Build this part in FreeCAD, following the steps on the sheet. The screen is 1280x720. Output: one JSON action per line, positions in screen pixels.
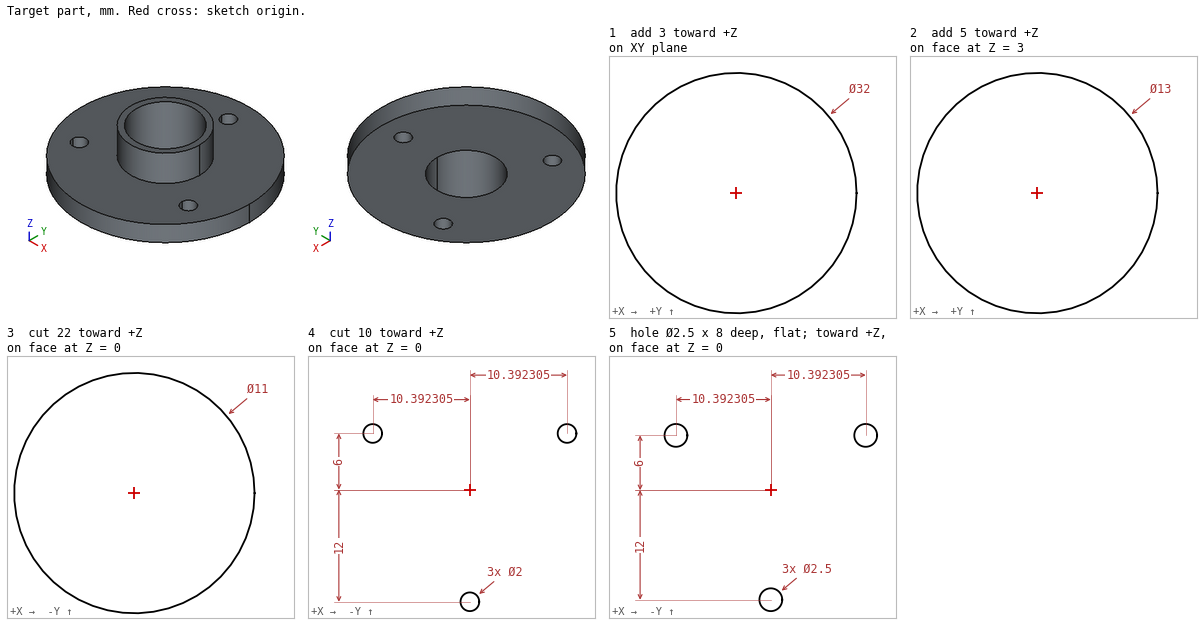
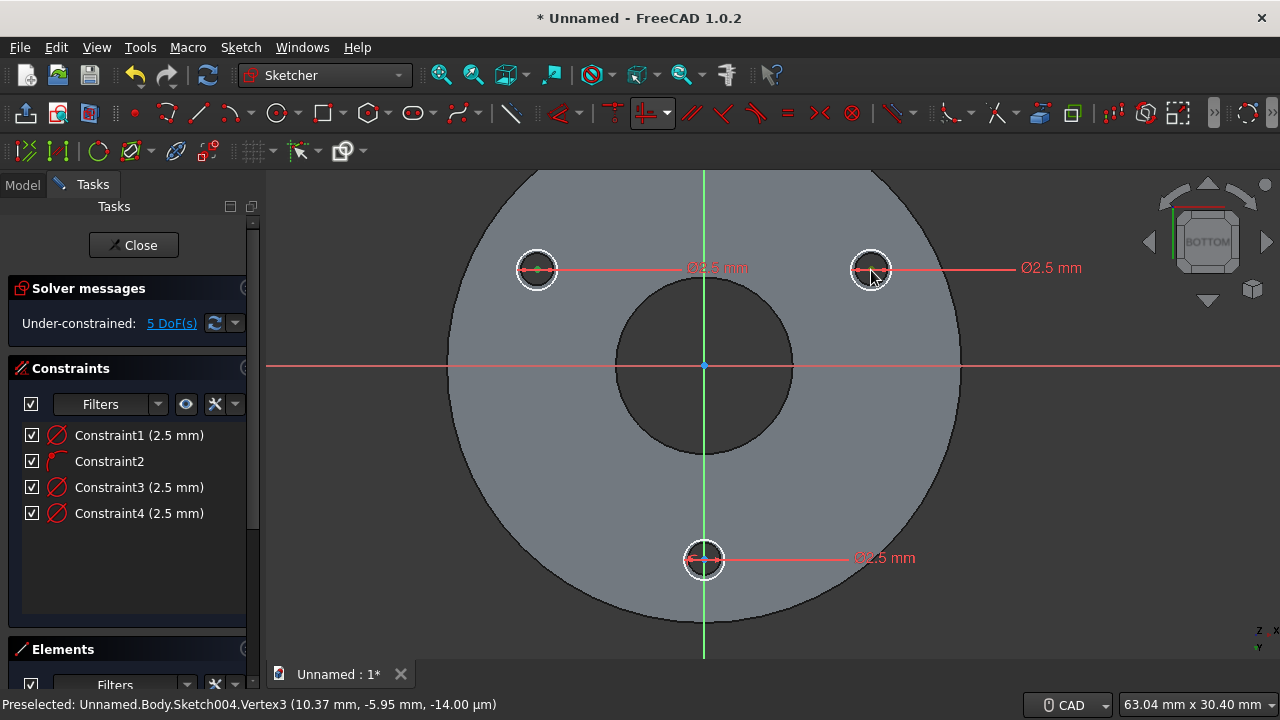
{"action": "key", "text": "h"}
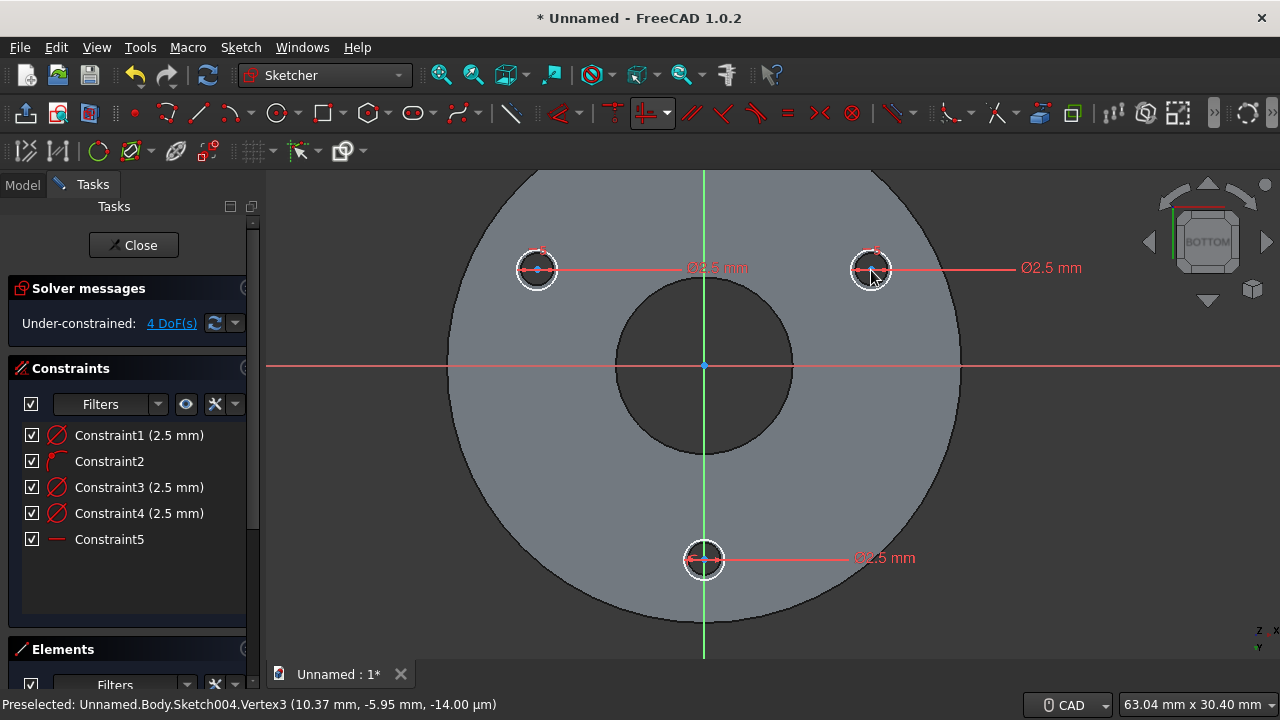
{"action": "left_click", "coordinate": [558, 114]}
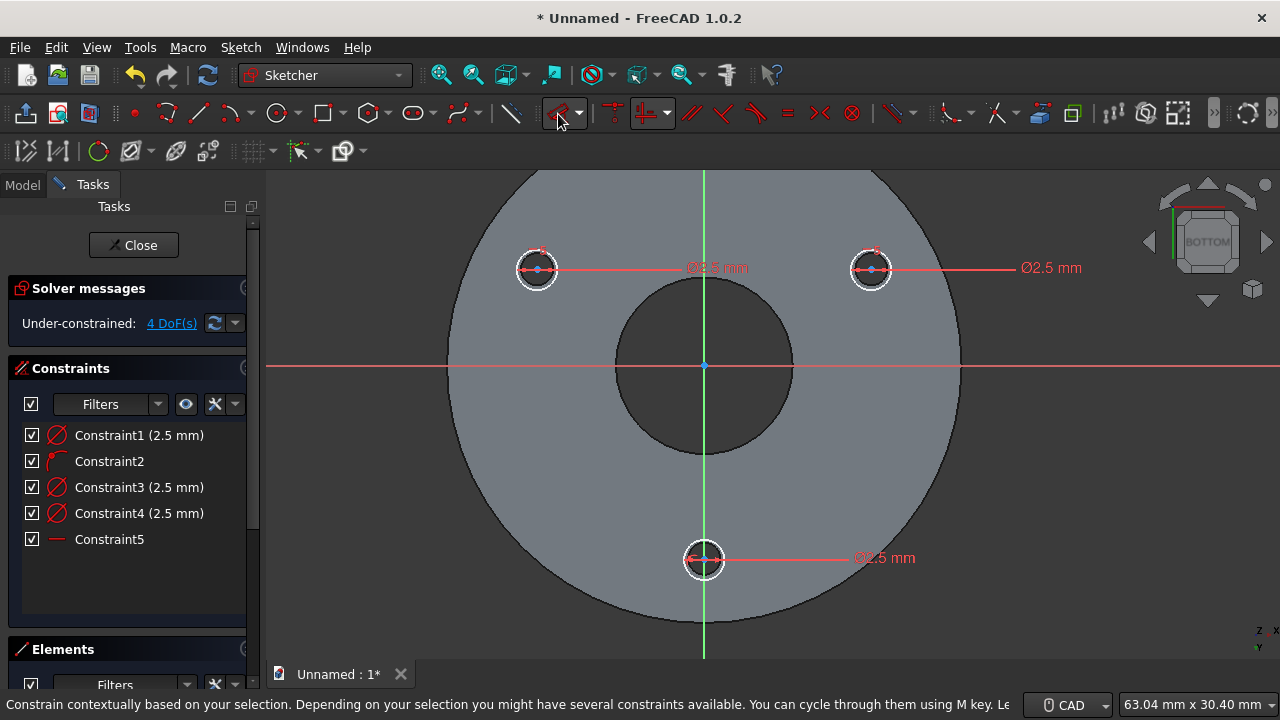
{"action": "left_click", "coordinate": [537, 270]}
{"action": "left_click", "coordinate": [503, 318]}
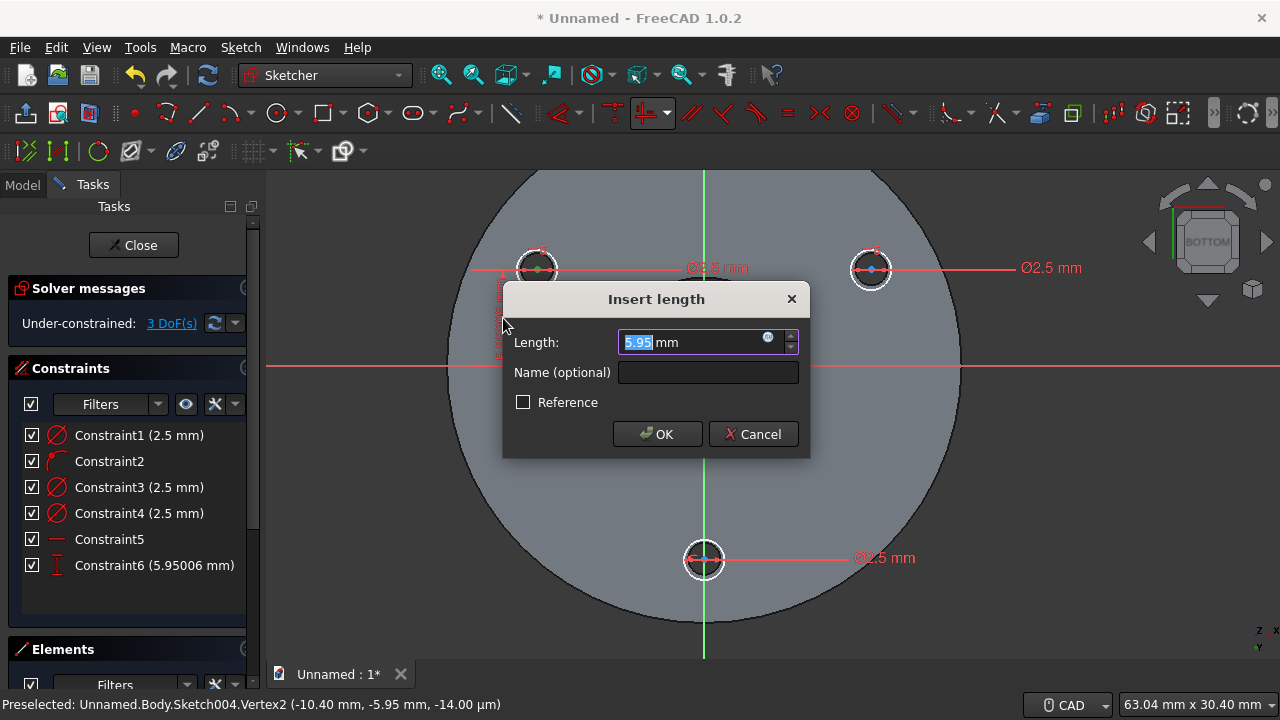
{"action": "type", "text": "6"}
{"action": "key", "text": "Return"}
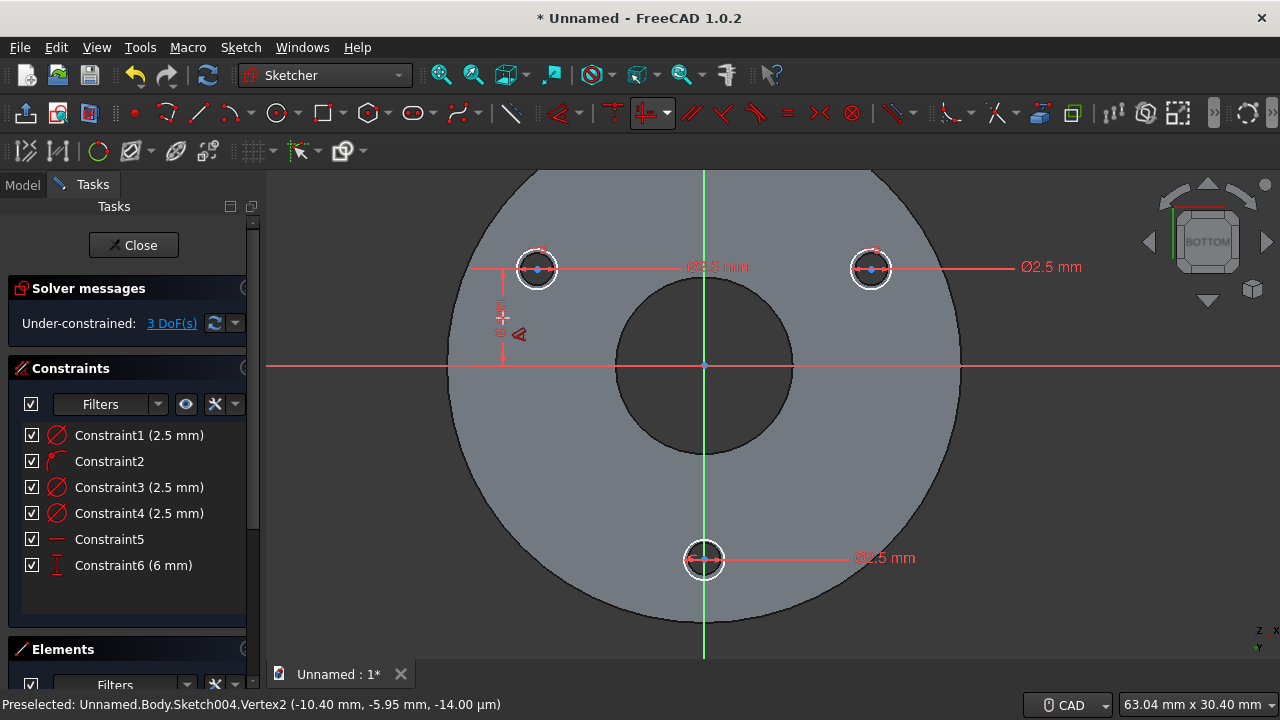
{"action": "left_click", "coordinate": [704, 560]}
{"action": "left_click", "coordinate": [738, 463]}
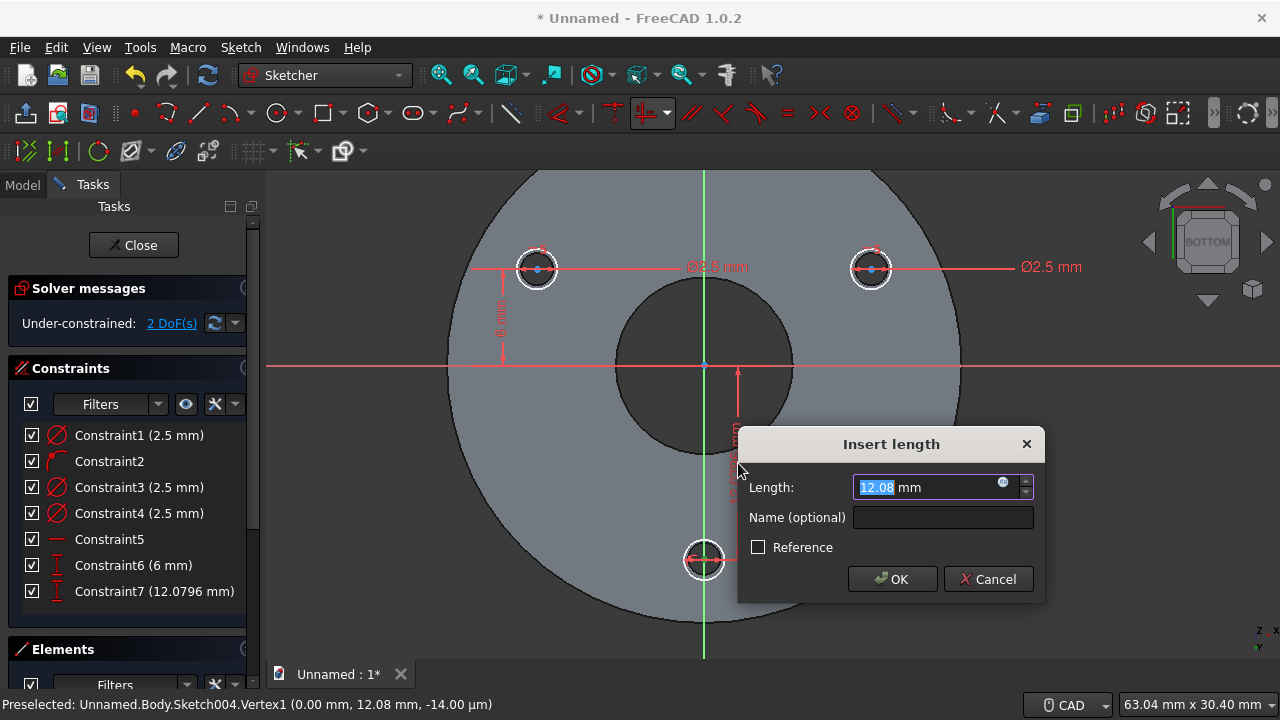
{"action": "type", "text": "12"}
{"action": "key", "text": "Return"}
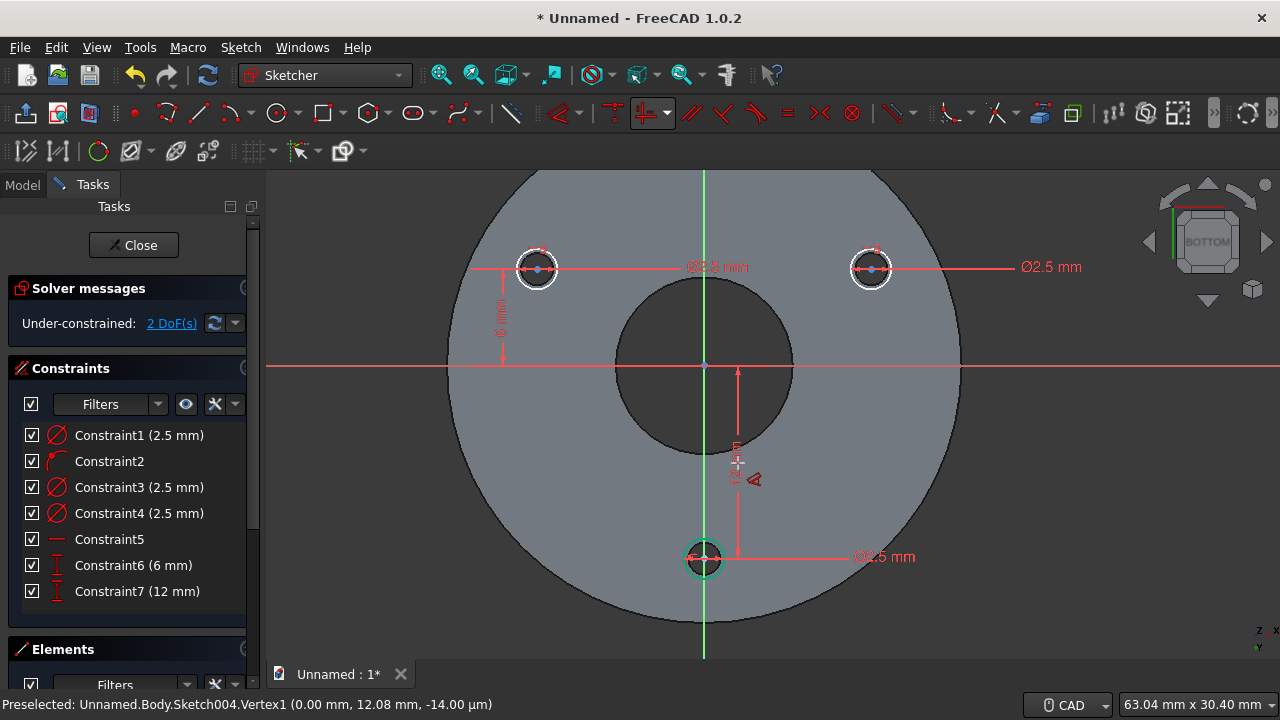
{"action": "left_click", "coordinate": [537, 269]}
{"action": "left_click", "coordinate": [621, 235]}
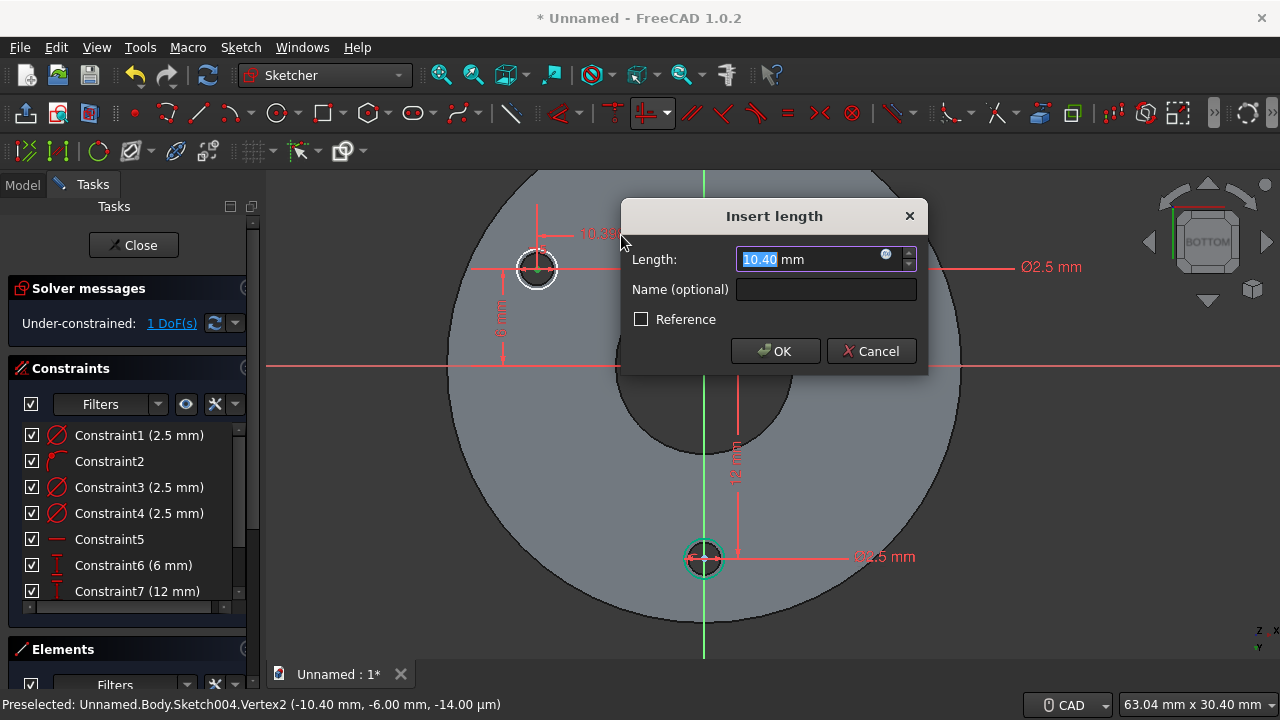
{"action": "type", "text": "10.392305"}
{"action": "key", "text": "Return"}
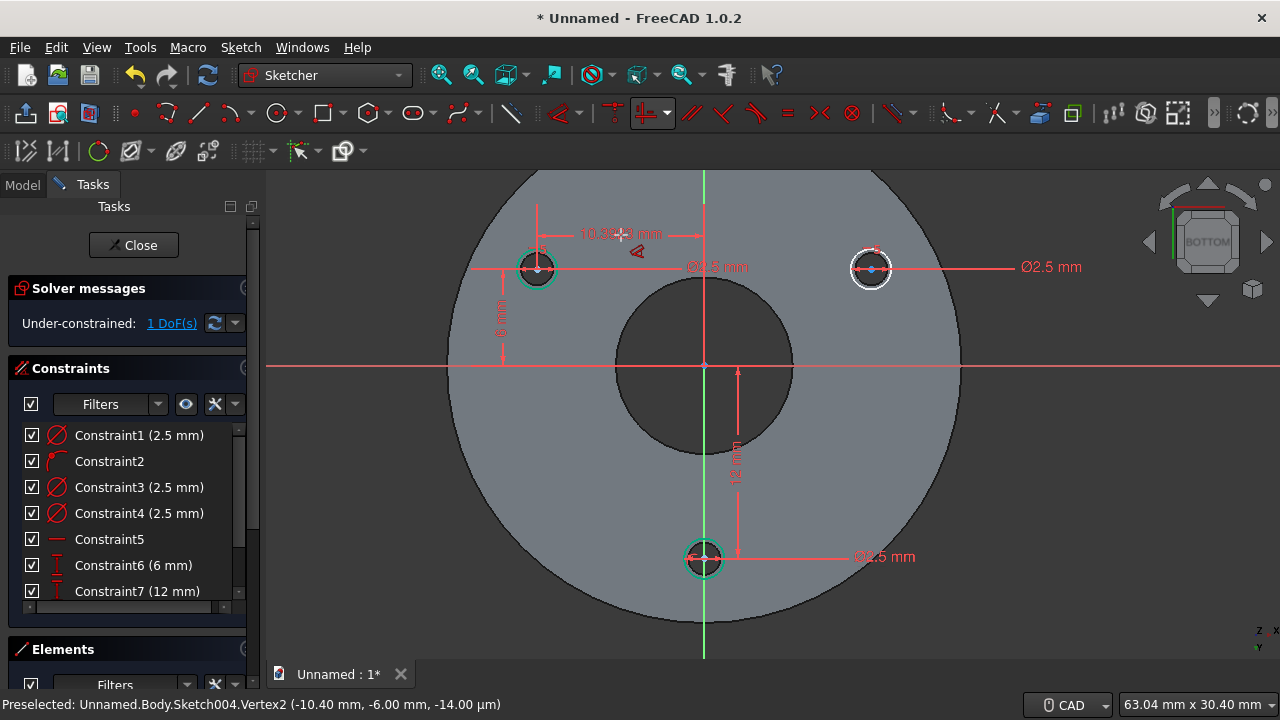
{"action": "left_click", "coordinate": [871, 269]}
{"action": "left_click", "coordinate": [788, 235]}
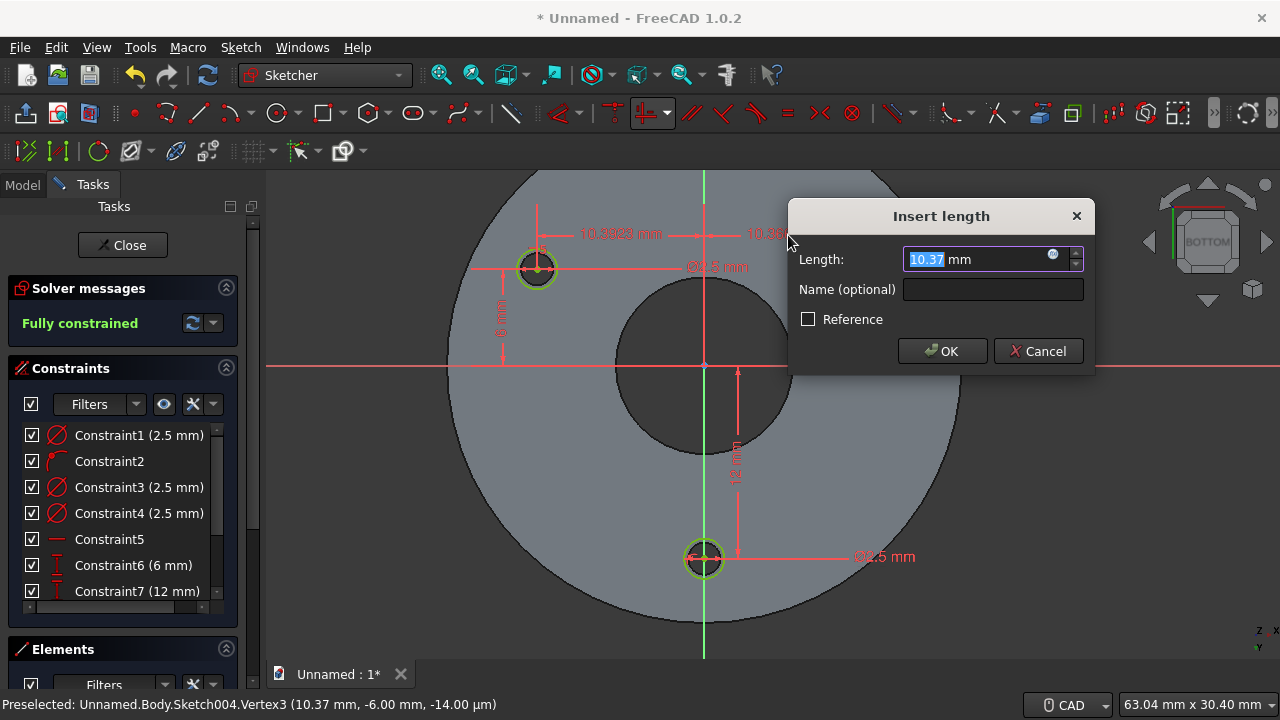
{"action": "type", "text": "10.392305"}
{"action": "key", "text": "Return"}
{"action": "key", "text": "Escape"}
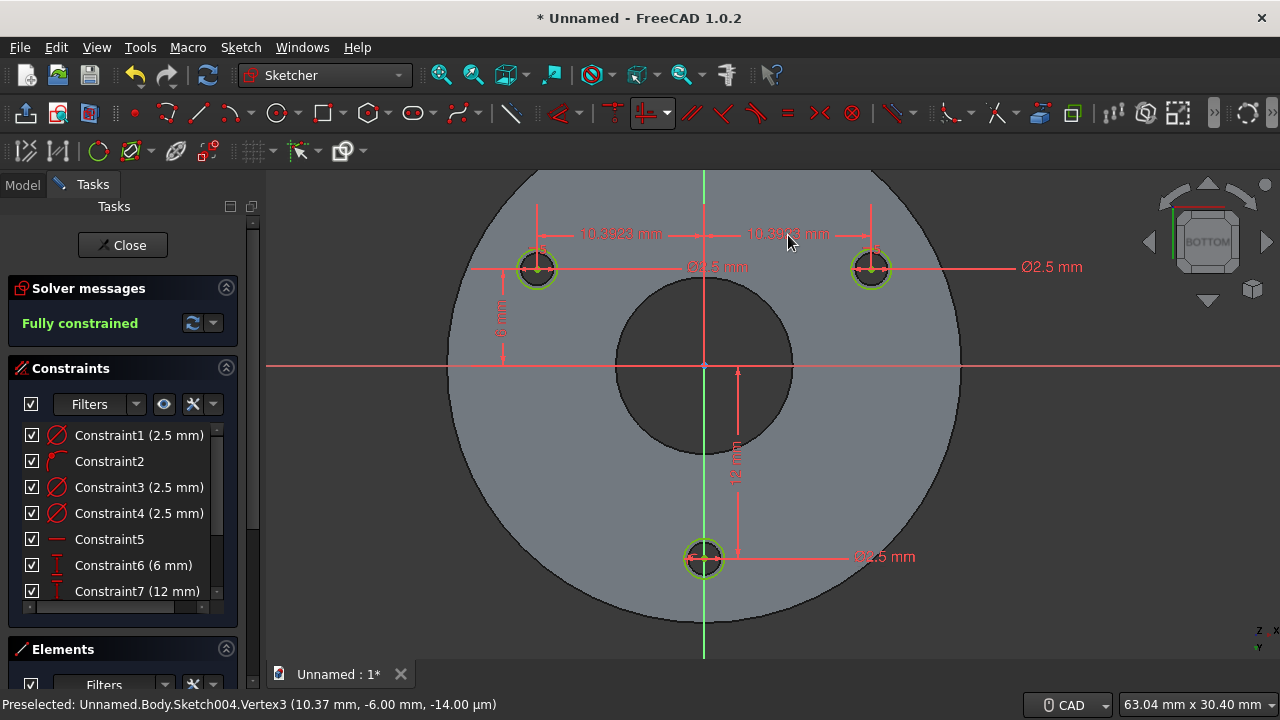
{"action": "left_click", "coordinate": [123, 245]}